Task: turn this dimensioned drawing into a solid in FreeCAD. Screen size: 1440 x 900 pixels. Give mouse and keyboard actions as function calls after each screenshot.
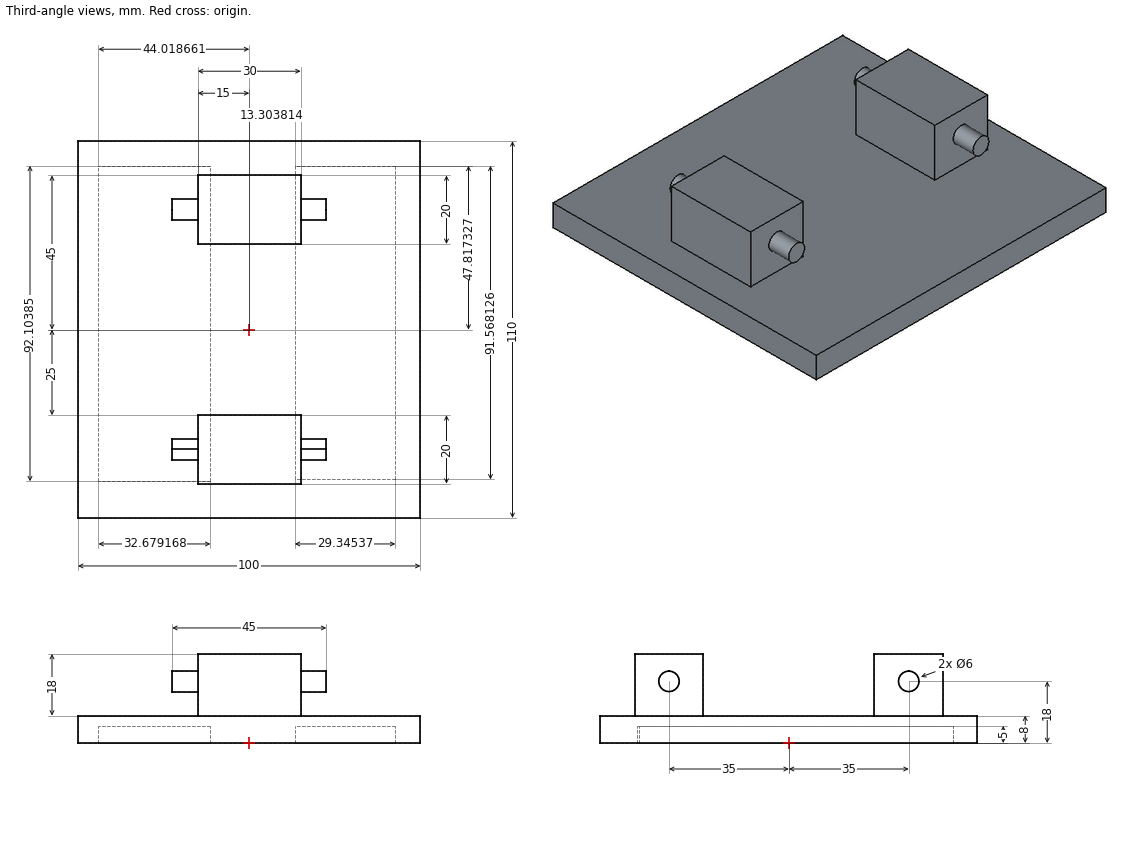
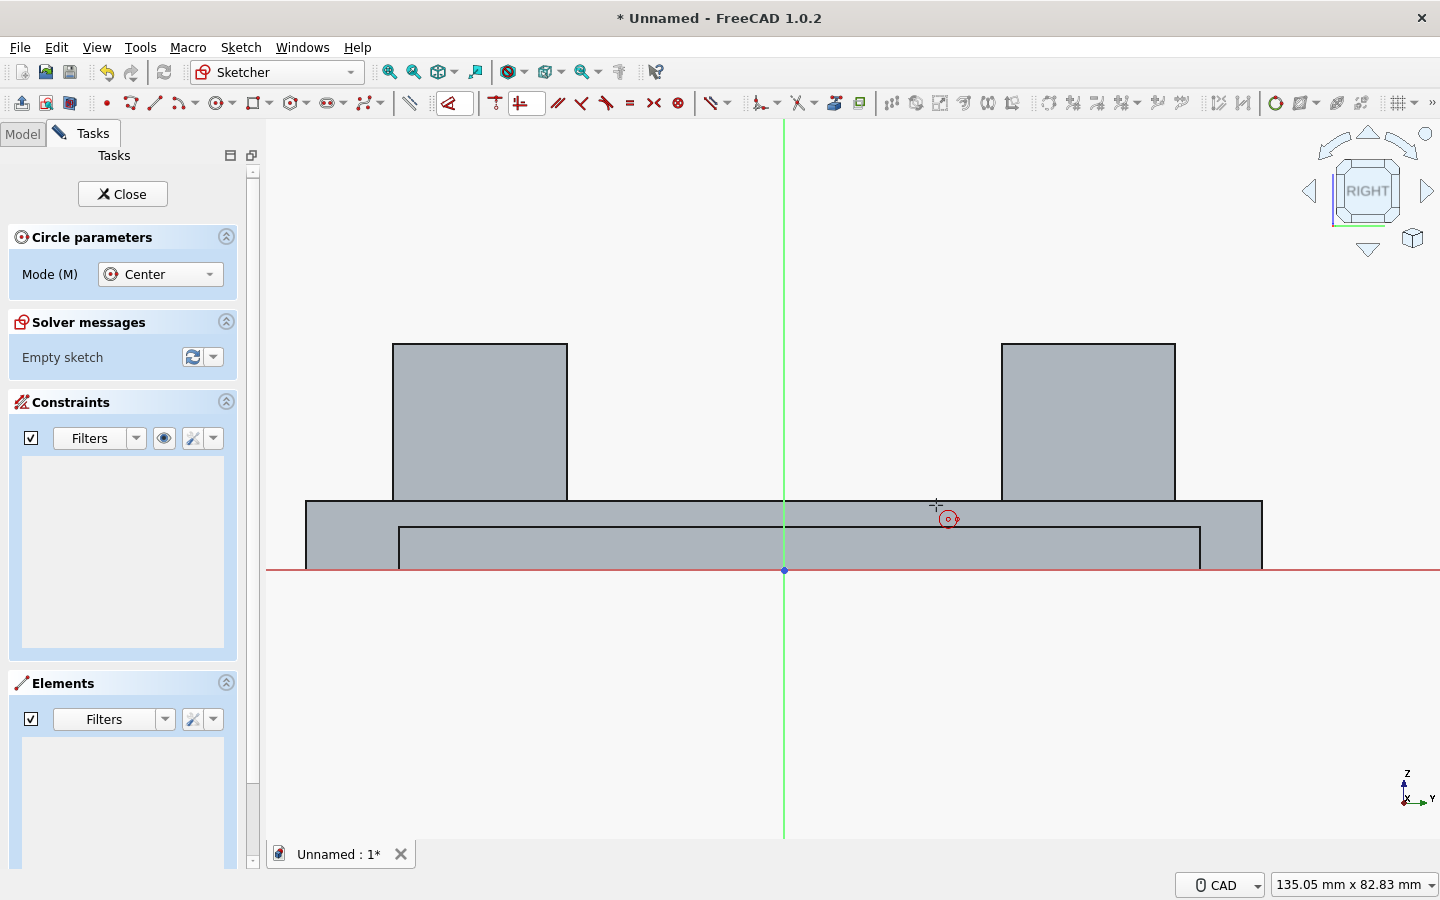
click(1089, 414)
move(1107, 395)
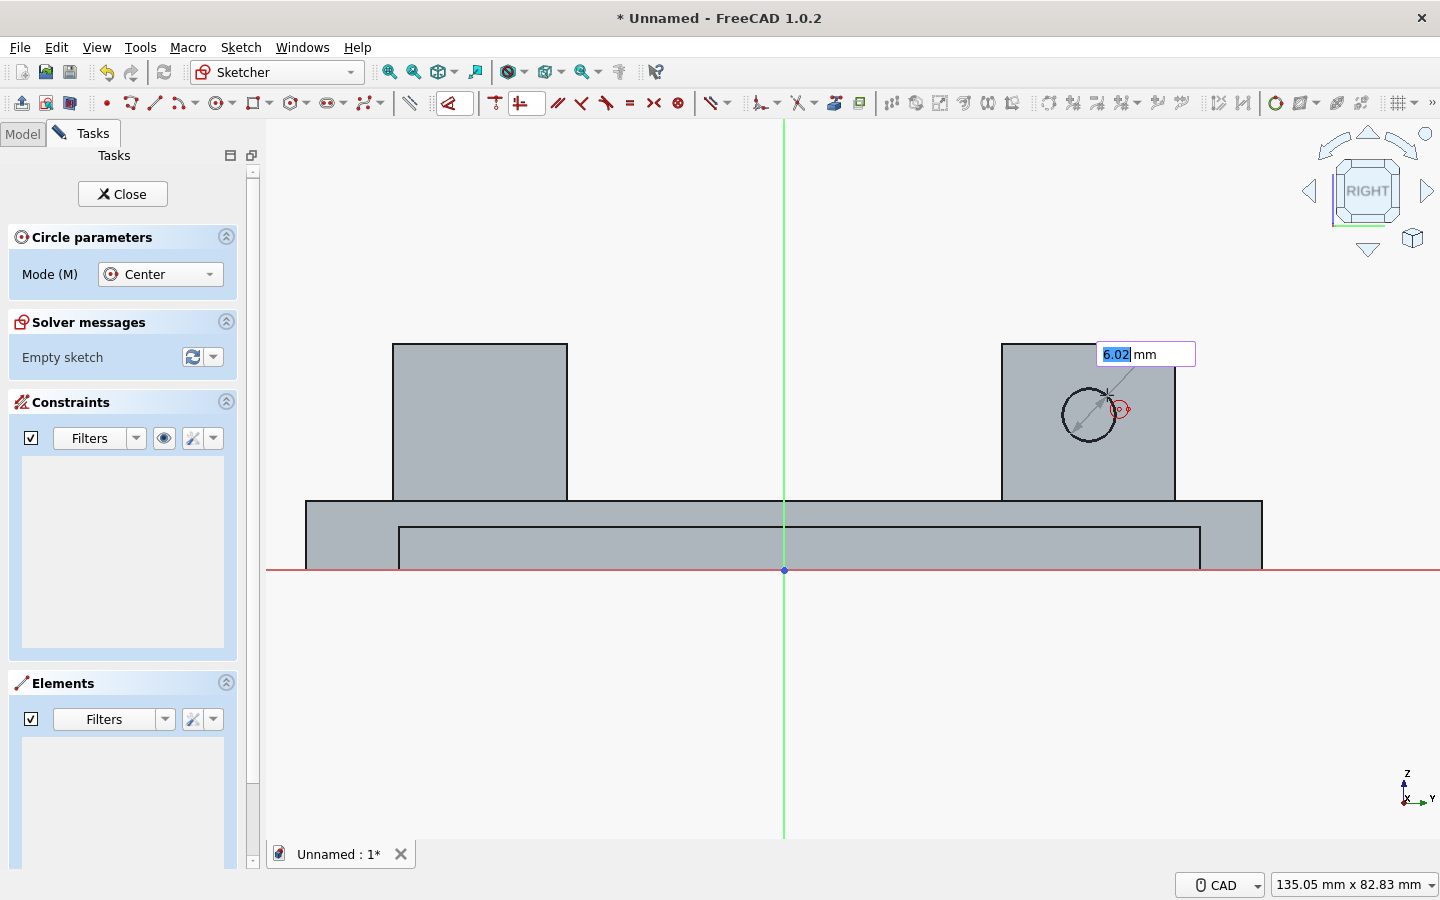
text(6)
key(Return)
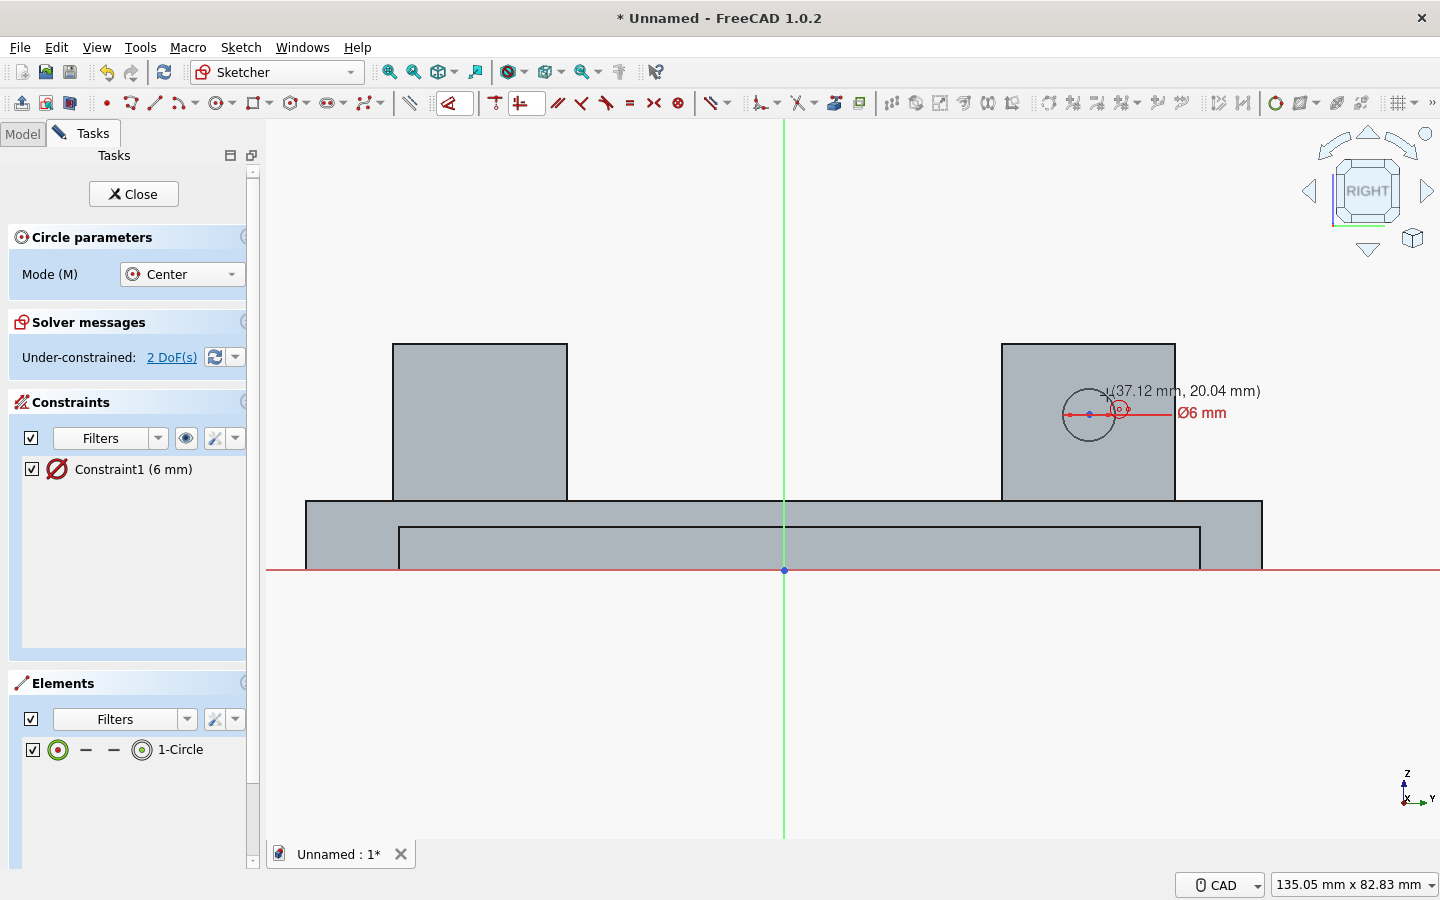
click(480, 414)
move(498, 395)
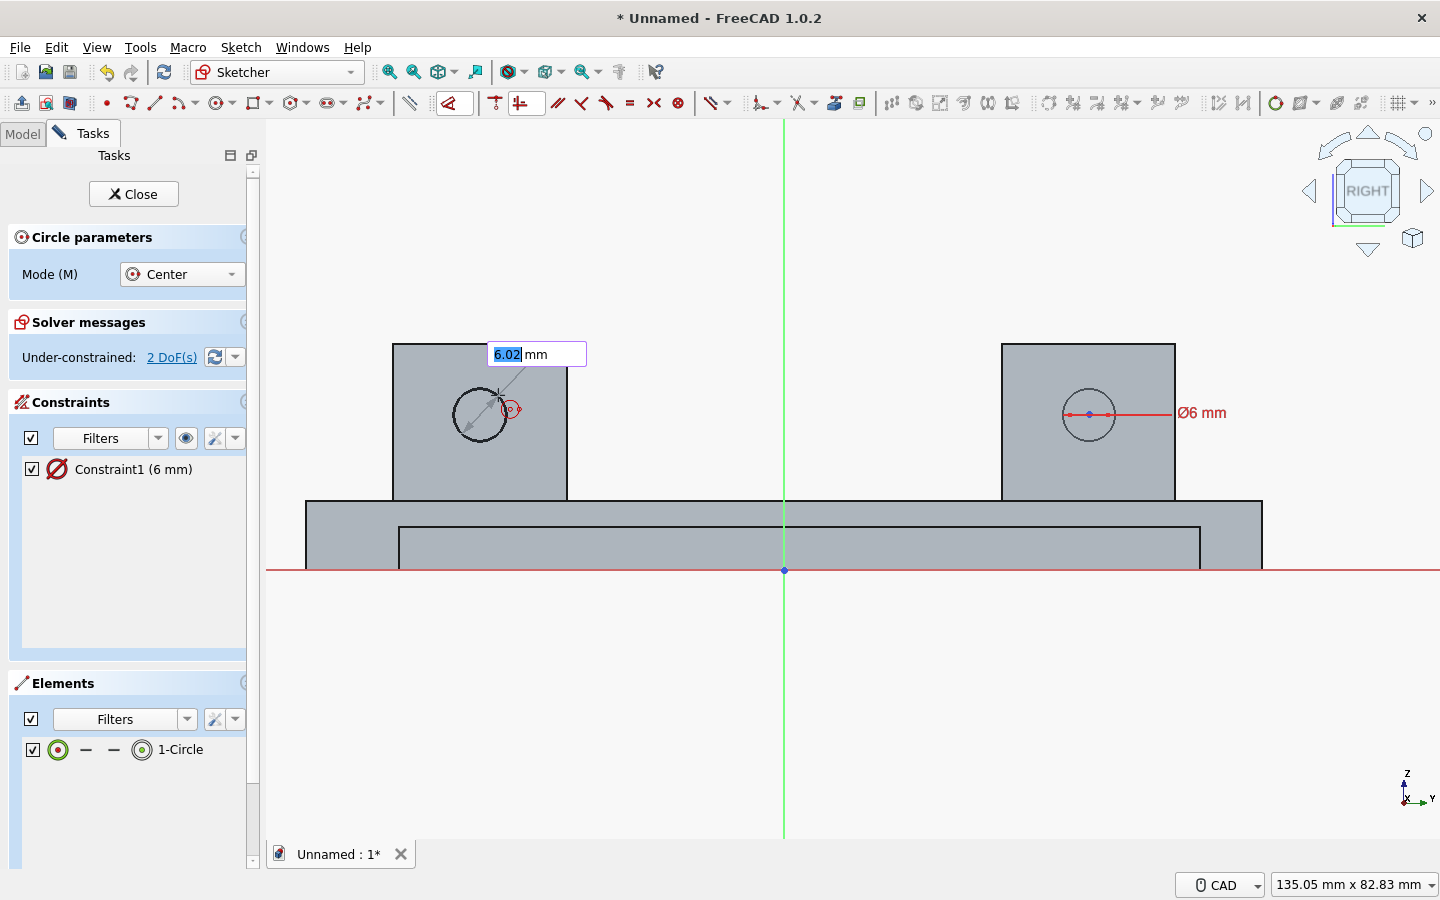
text(6)
key(Return)
key(Escape)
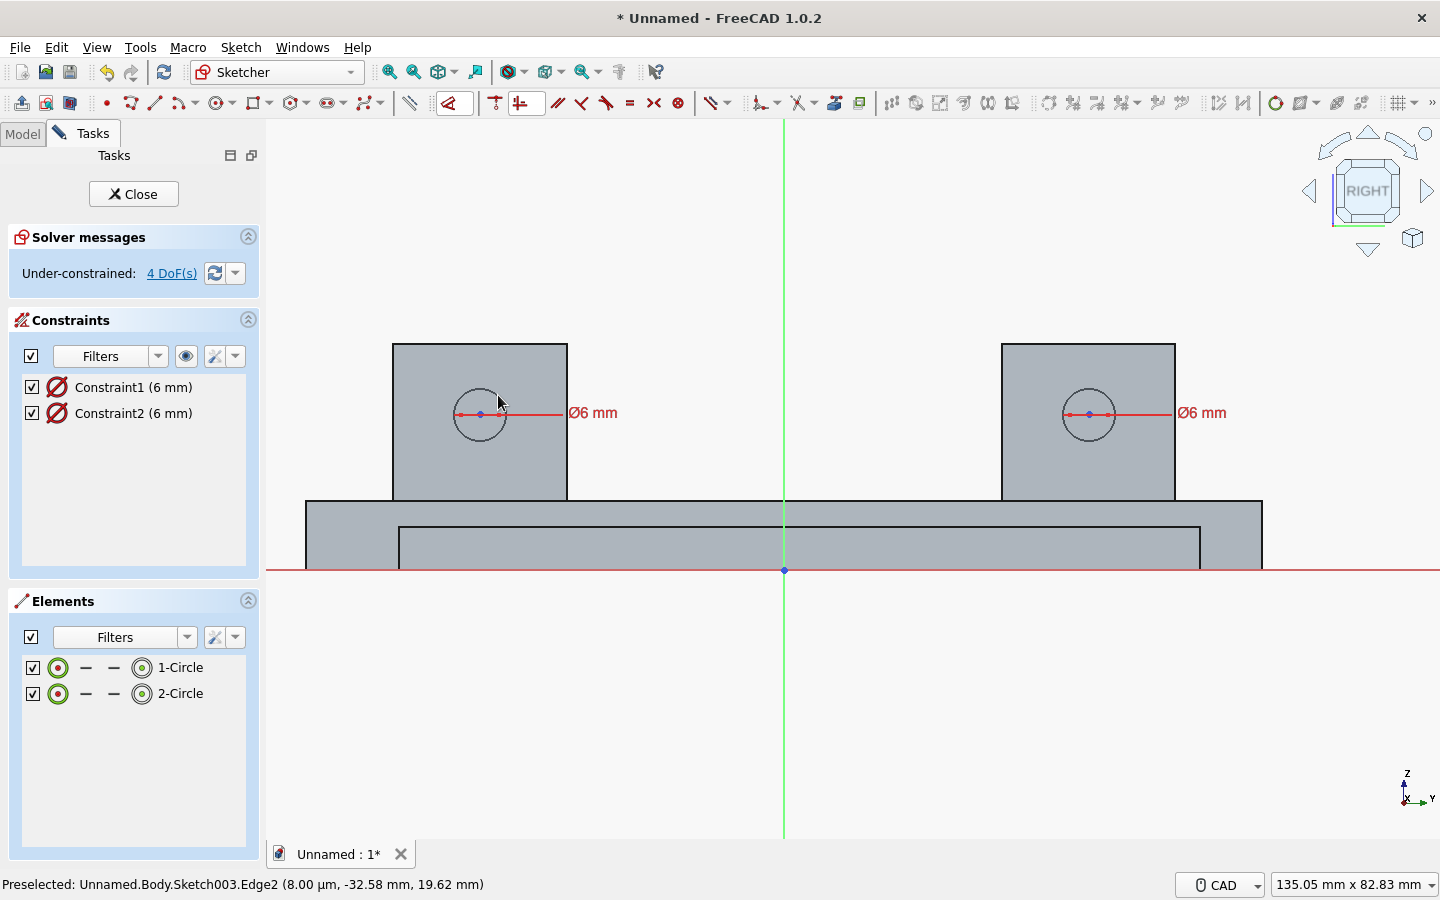
click(1089, 415)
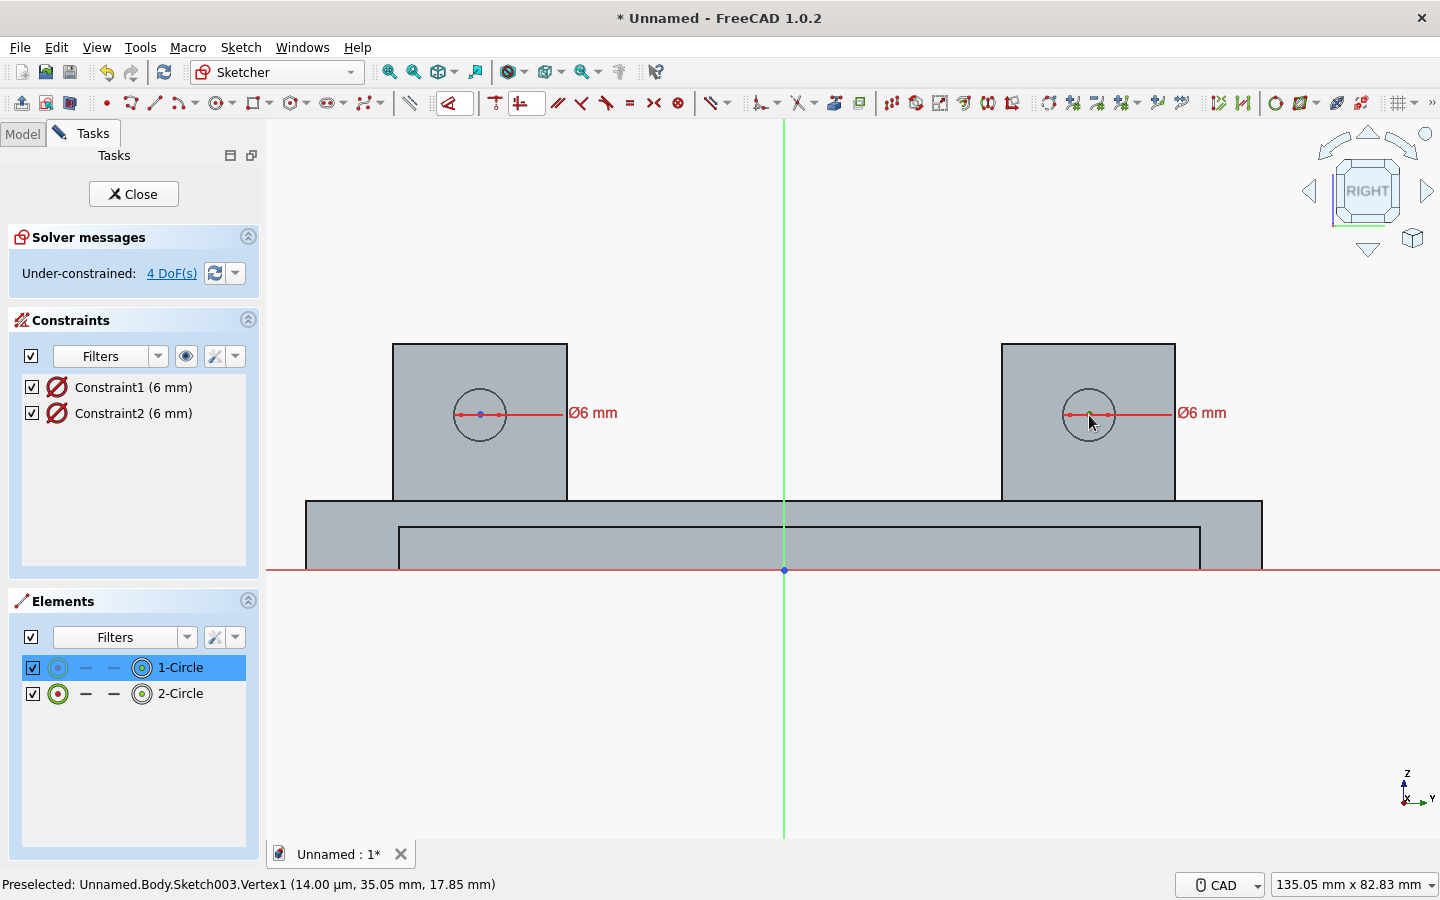
click(480, 415)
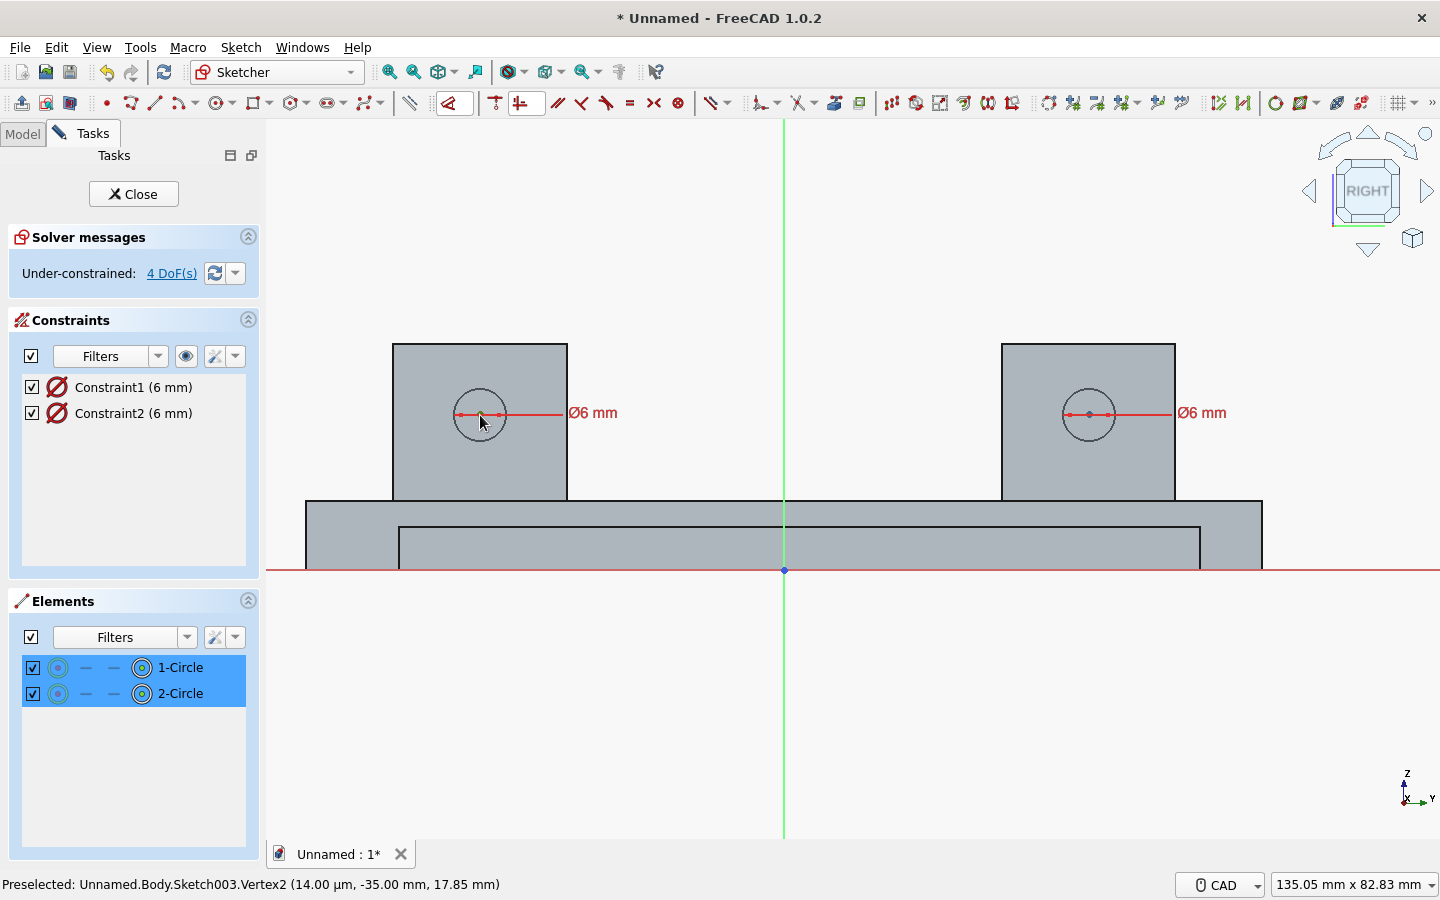
key(h)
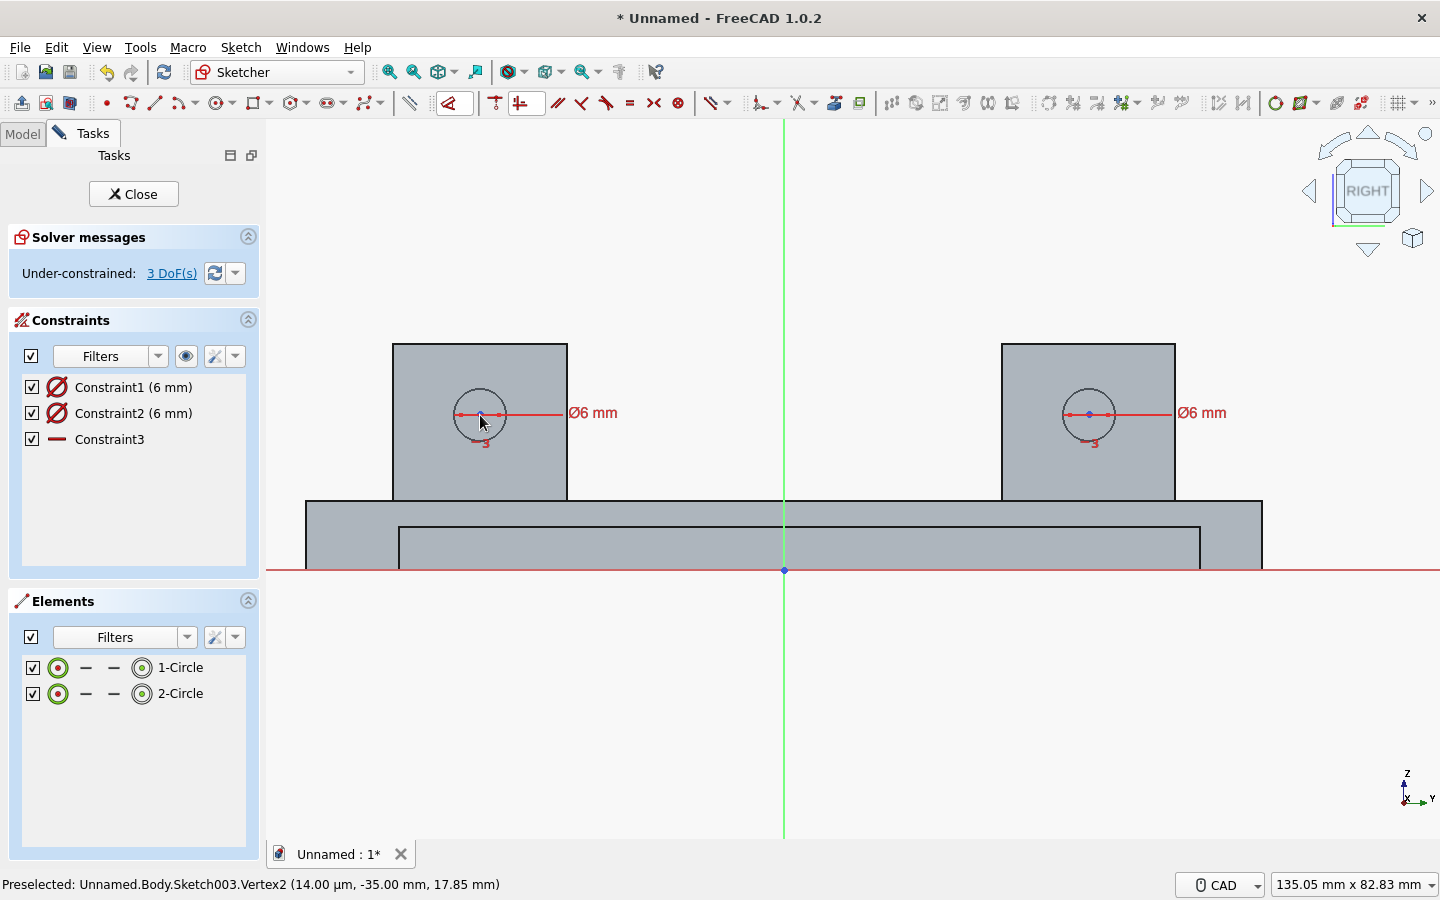
click(448, 104)